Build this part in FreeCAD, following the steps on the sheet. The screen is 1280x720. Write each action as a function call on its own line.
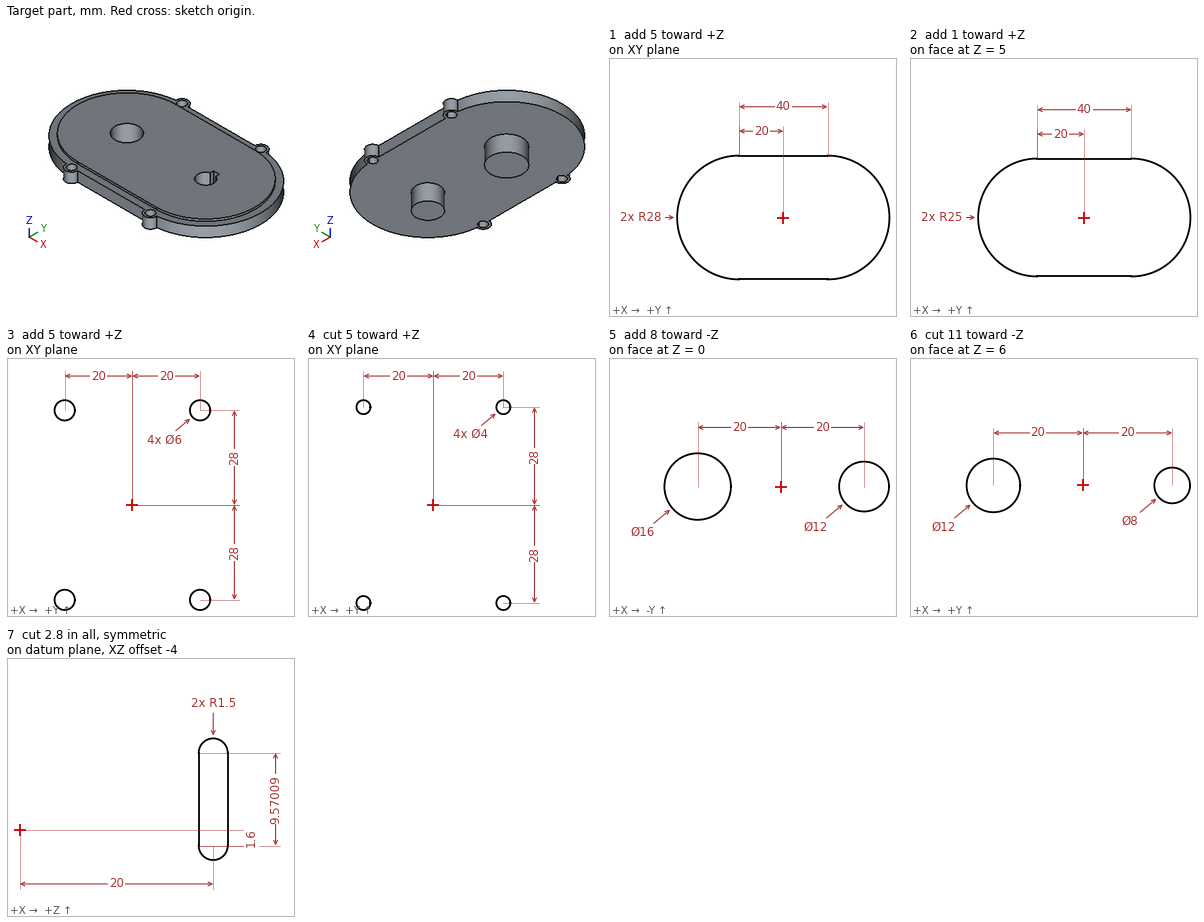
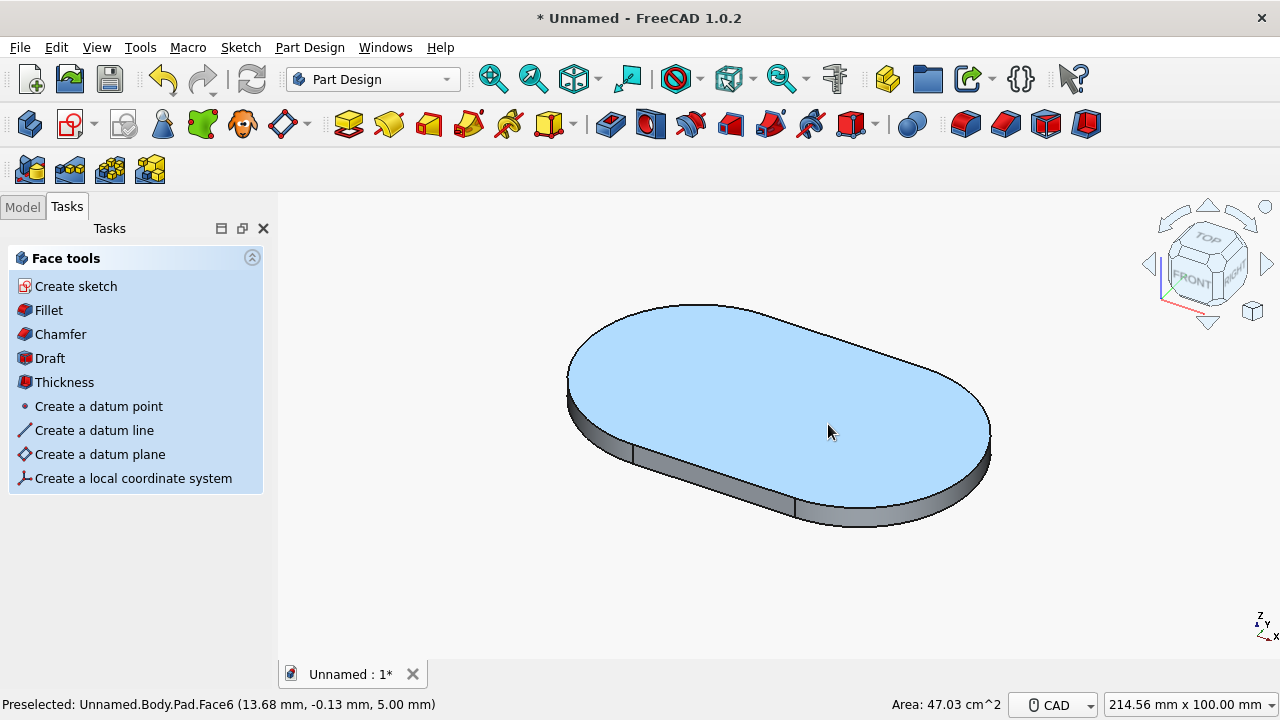
click(70, 124)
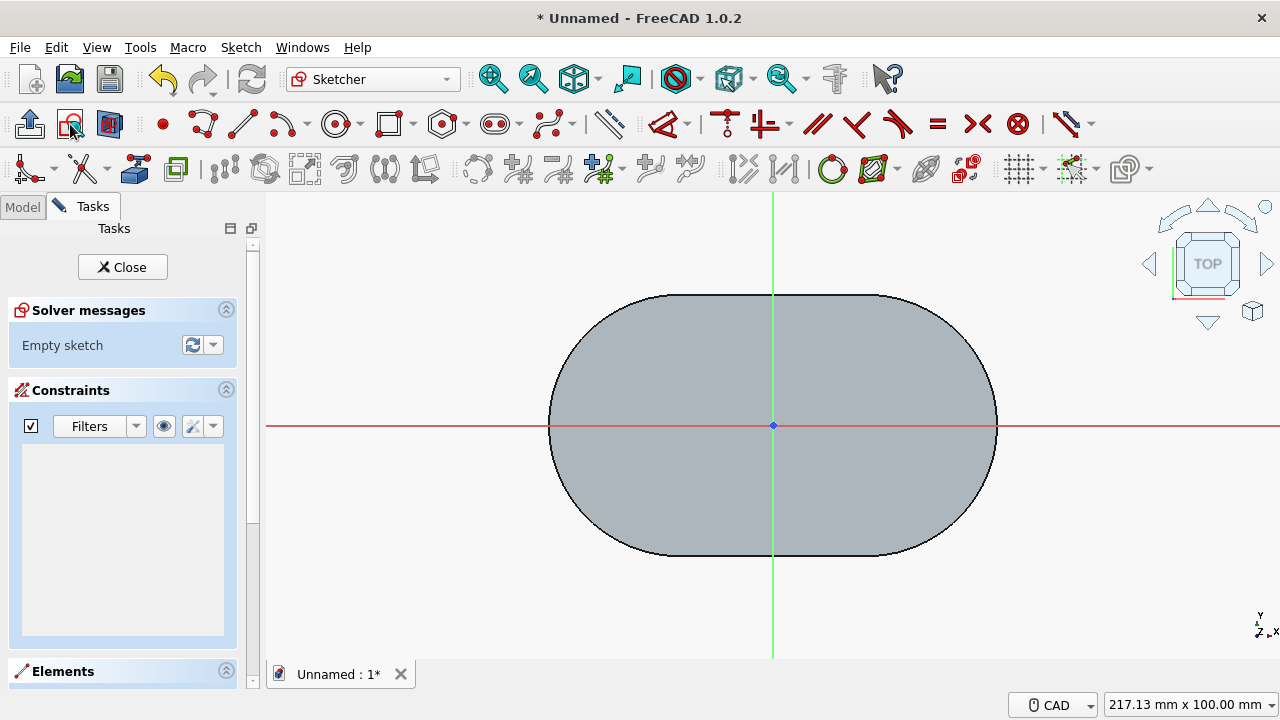
click(496, 124)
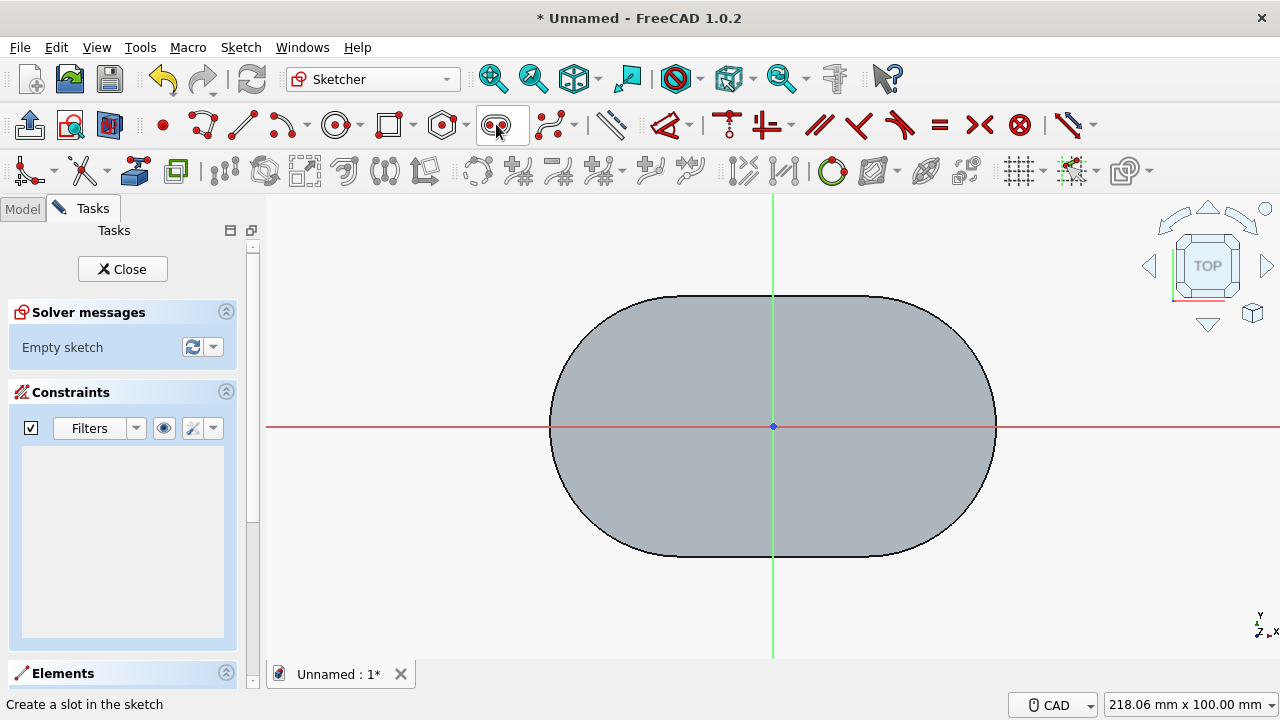
click(680, 426)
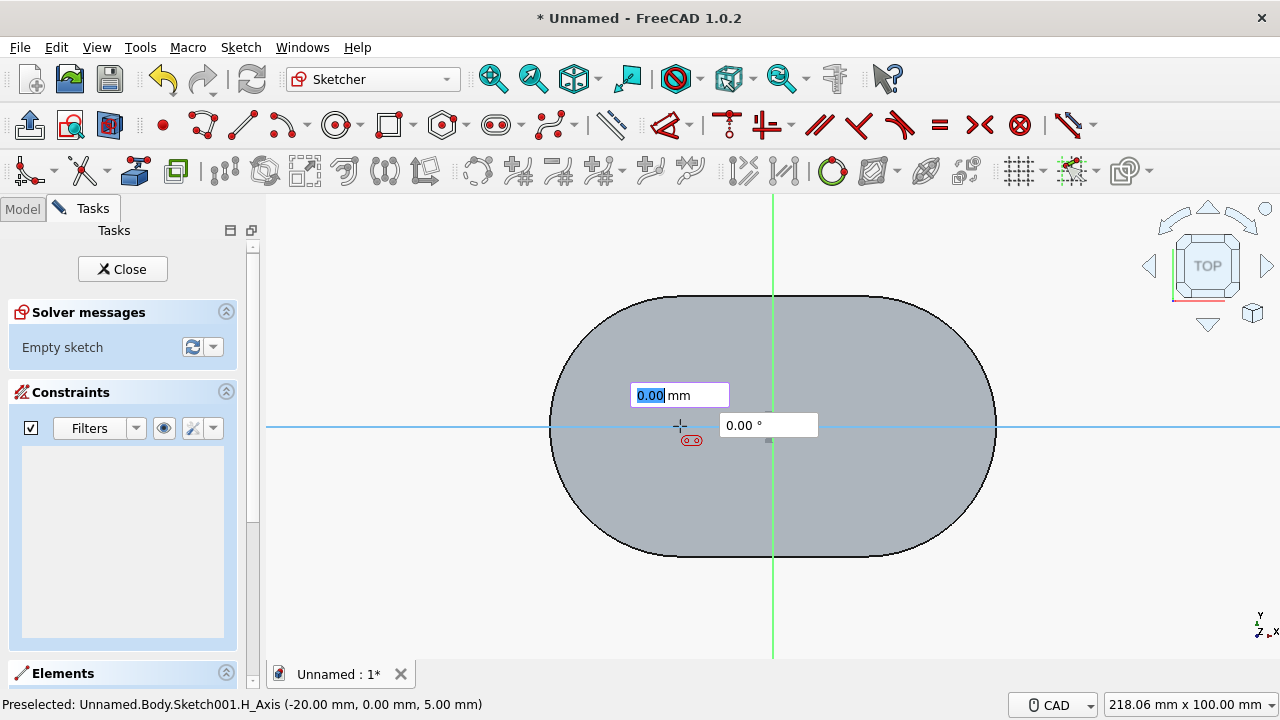
click(866, 418)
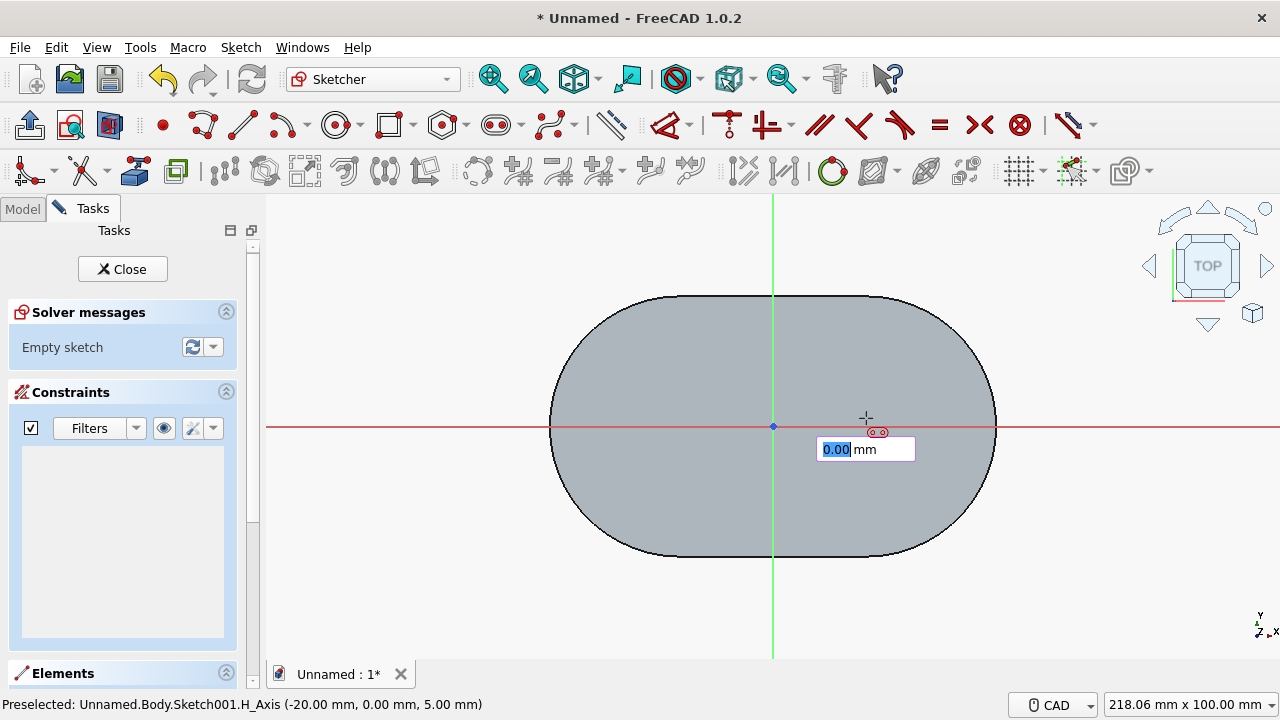
click(801, 310)
key(Escape)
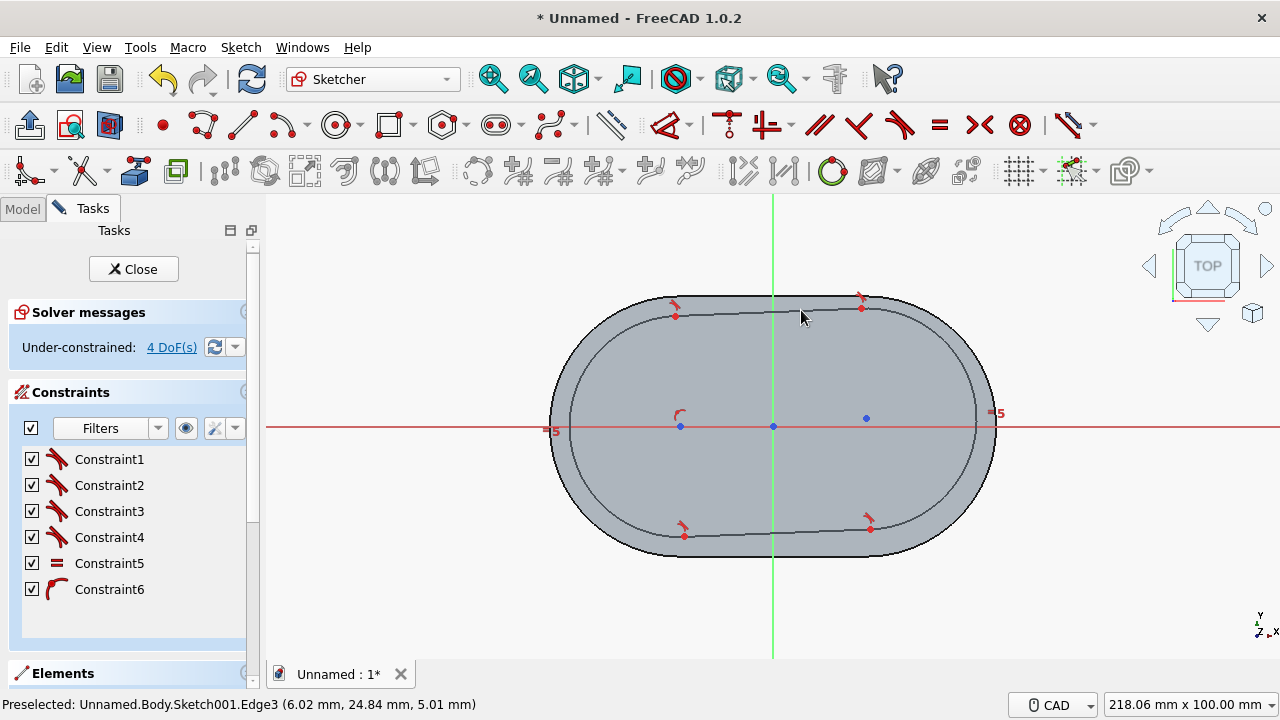
click(731, 314)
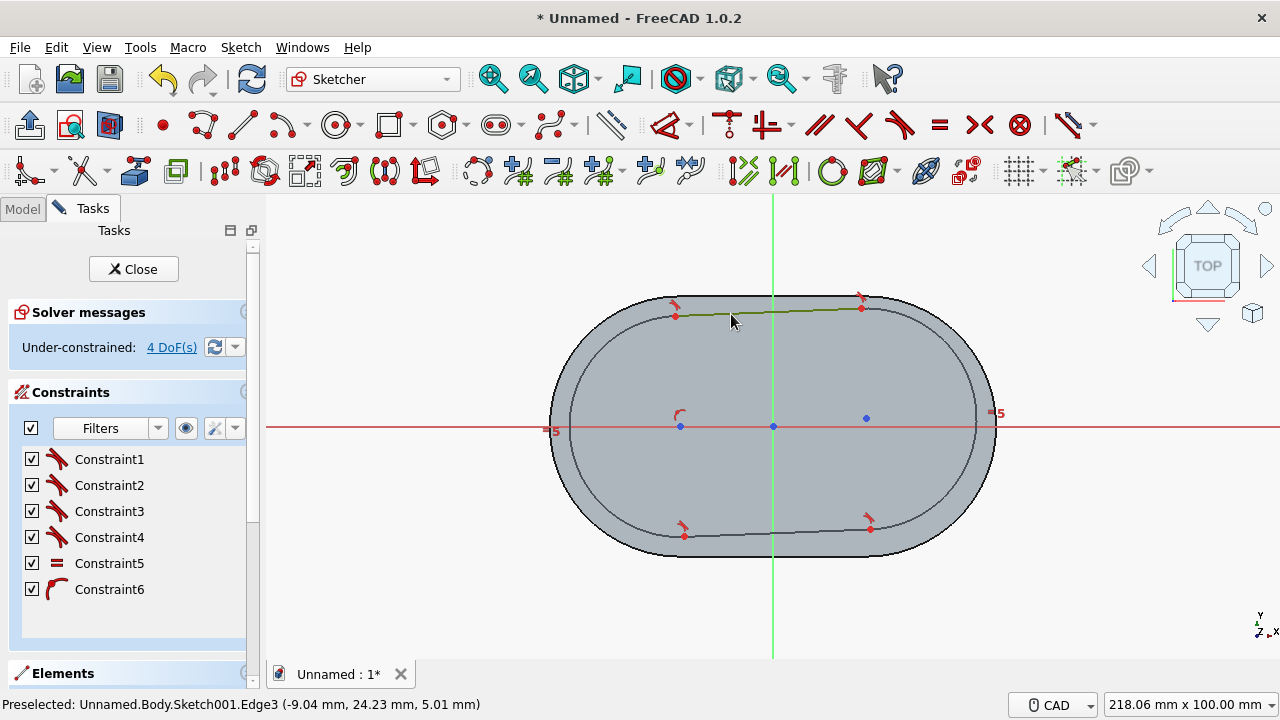
key(h)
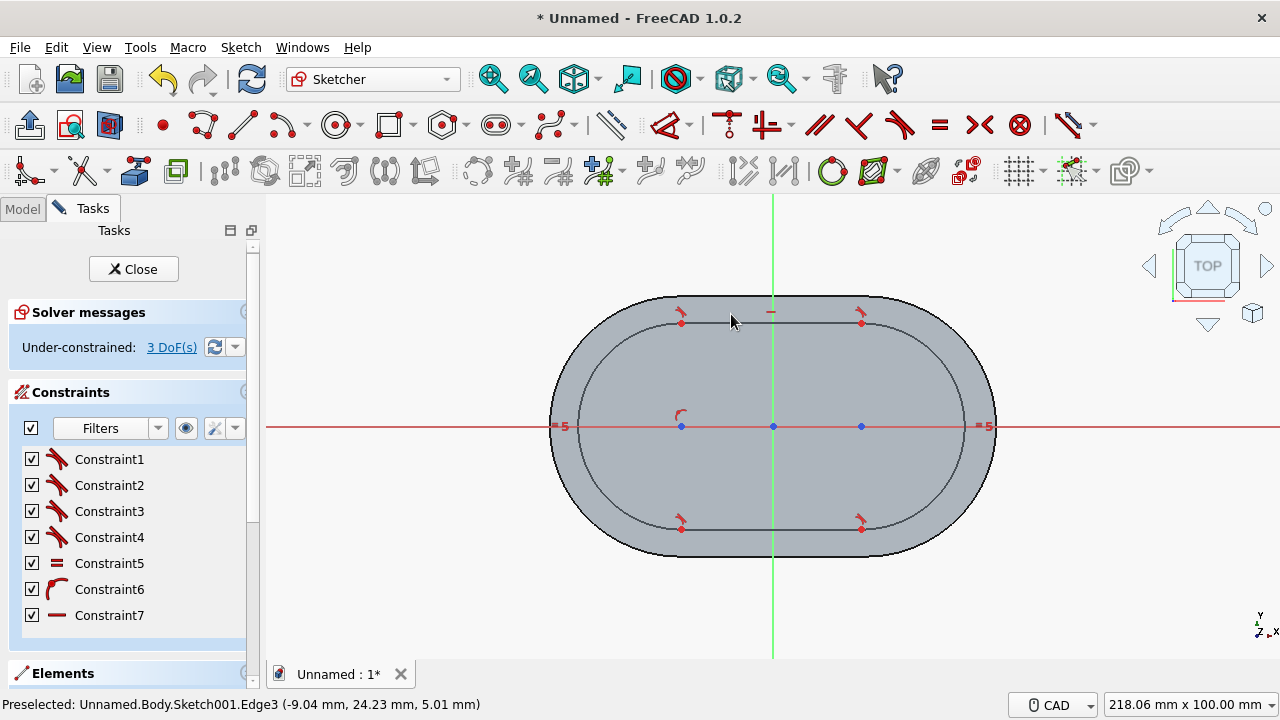
key(d)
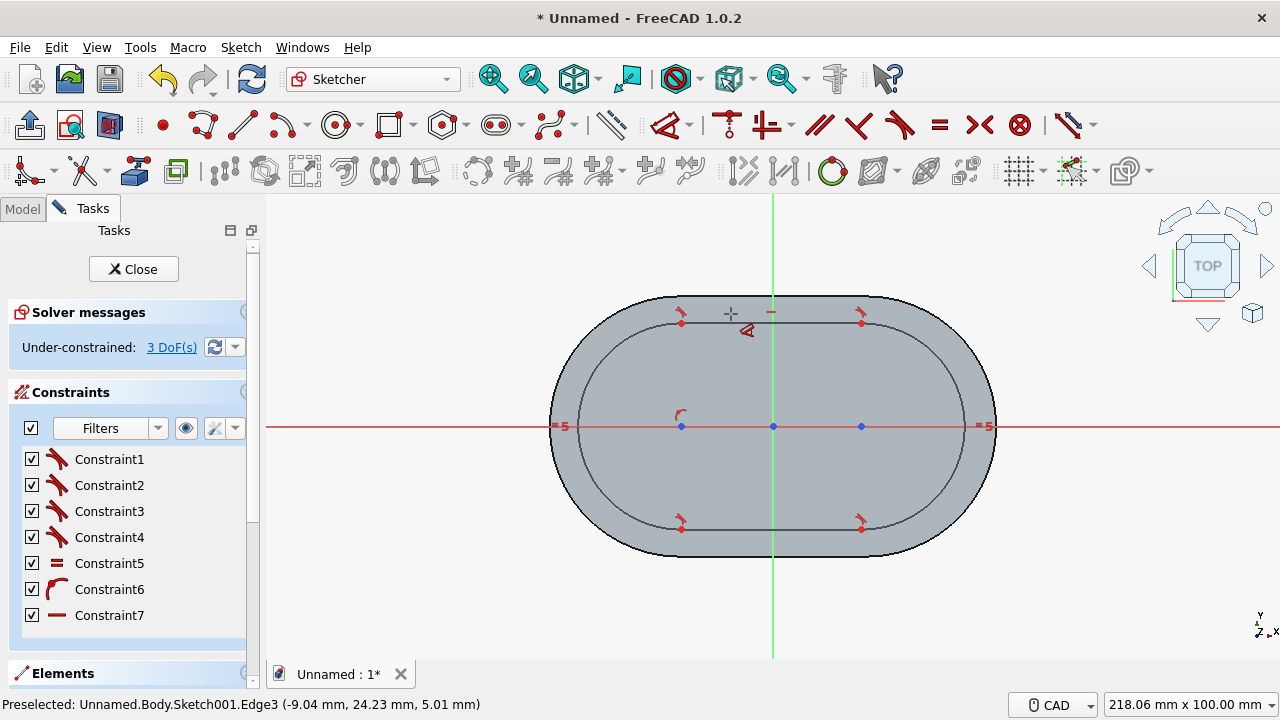
click(598, 366)
click(572, 347)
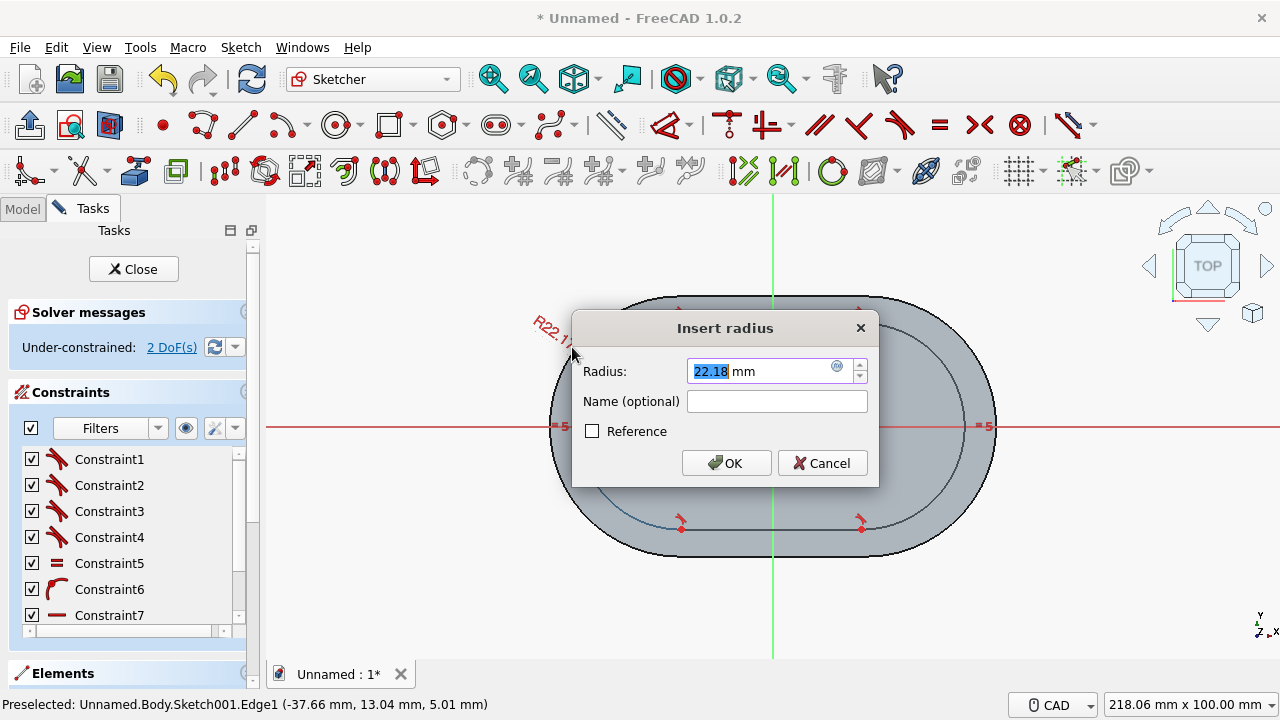
text(25)
key(Return)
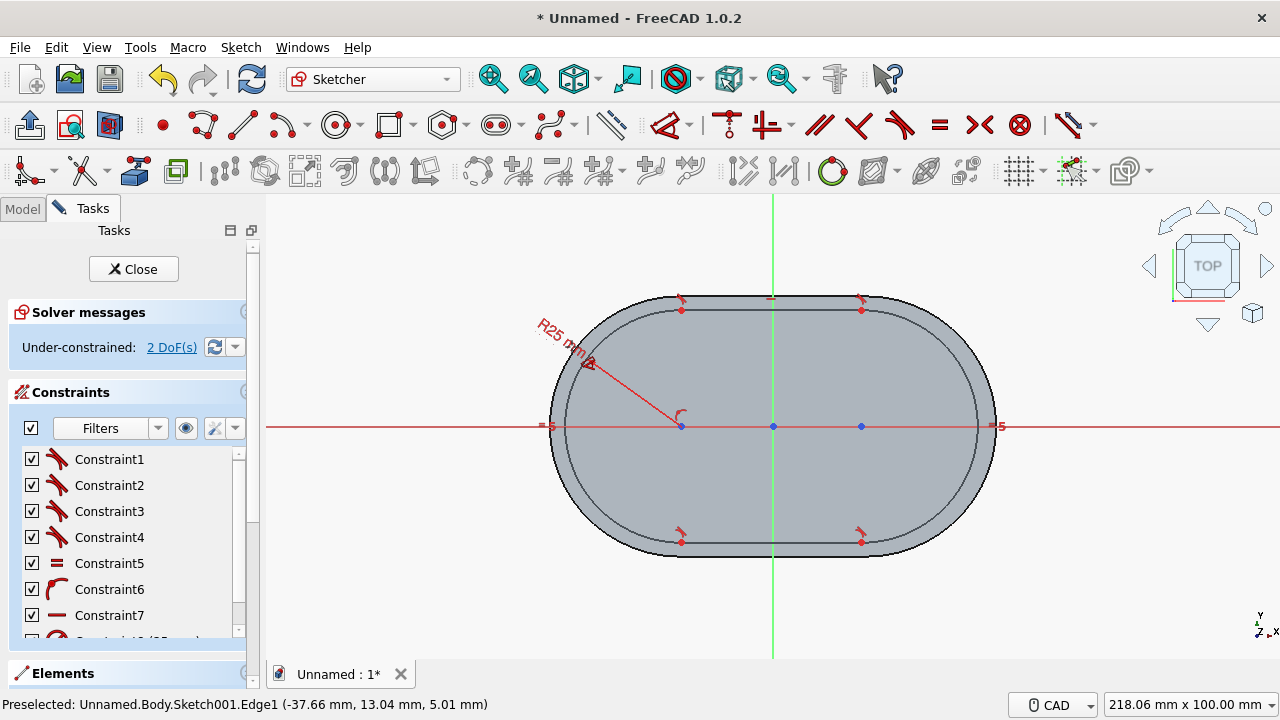
click(735, 310)
click(730, 276)